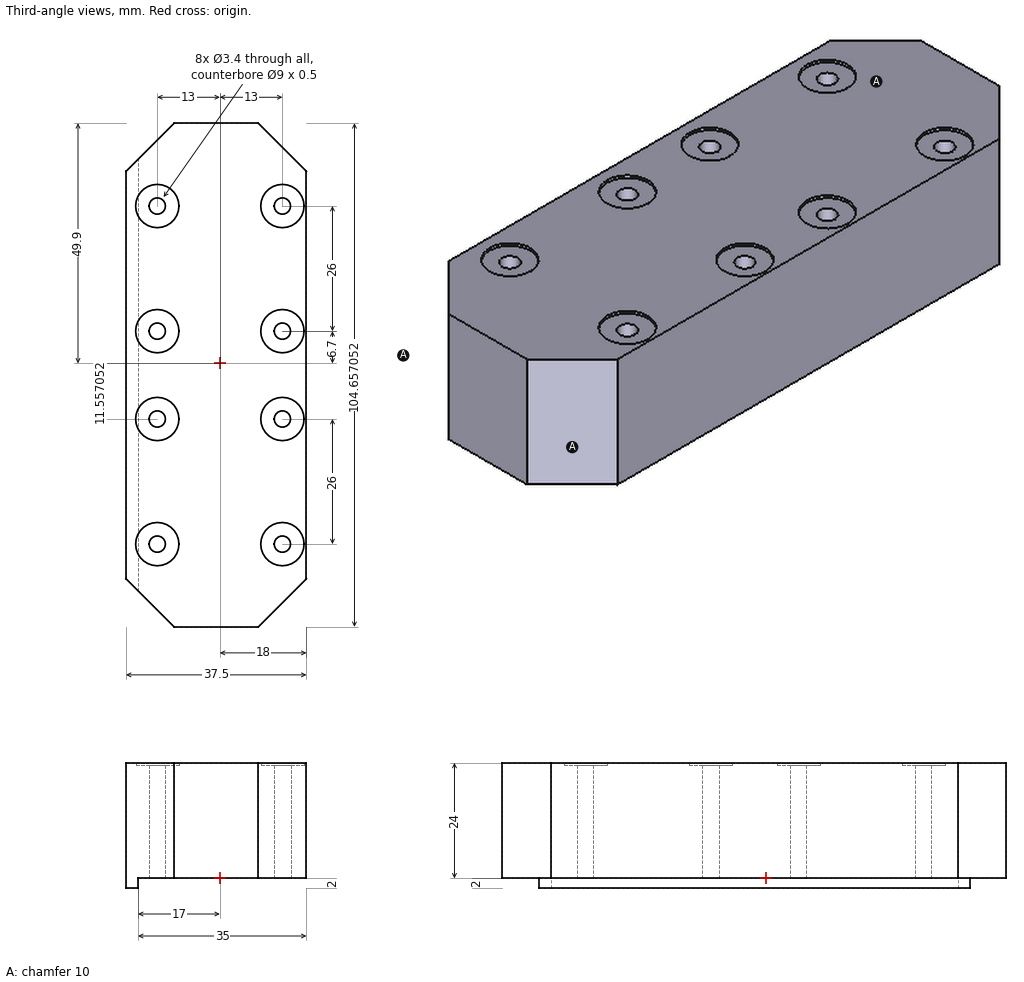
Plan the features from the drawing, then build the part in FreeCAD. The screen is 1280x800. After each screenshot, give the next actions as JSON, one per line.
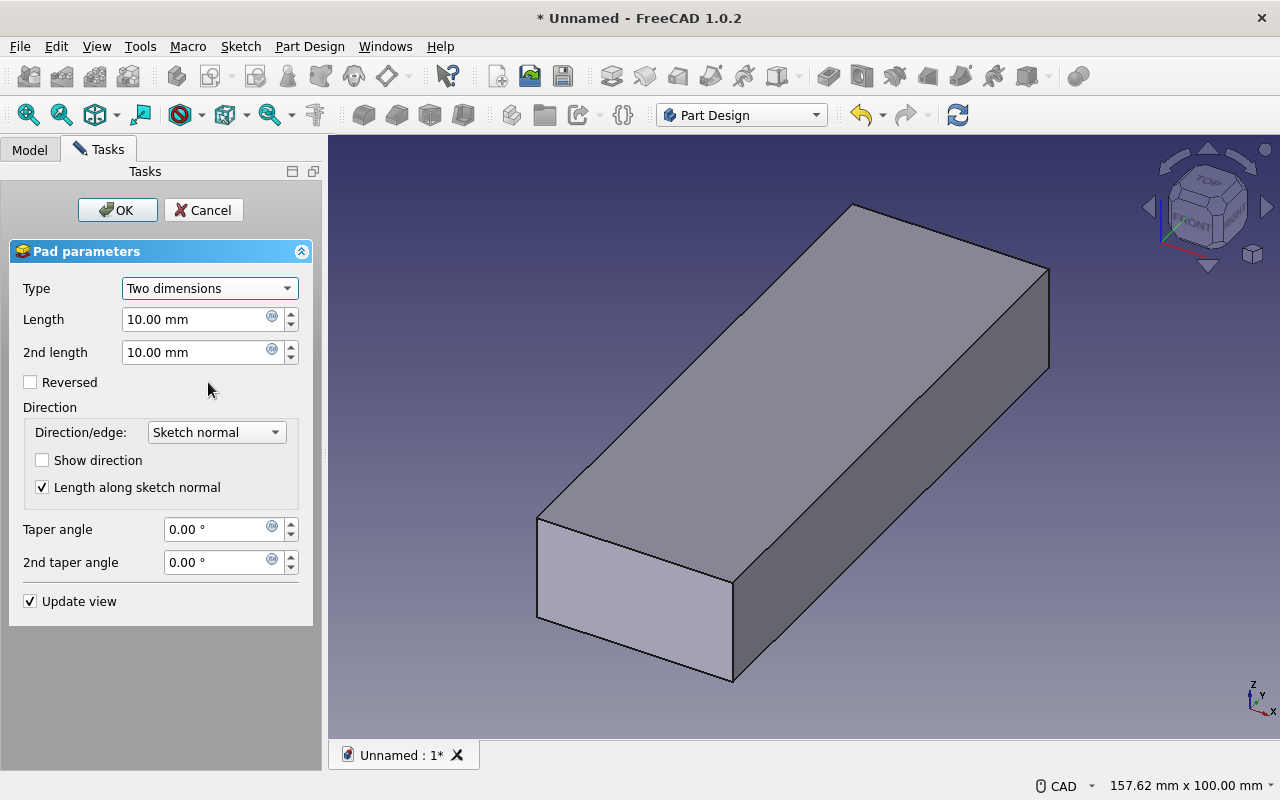
{"action": "triple_click", "coordinate": [204, 320]}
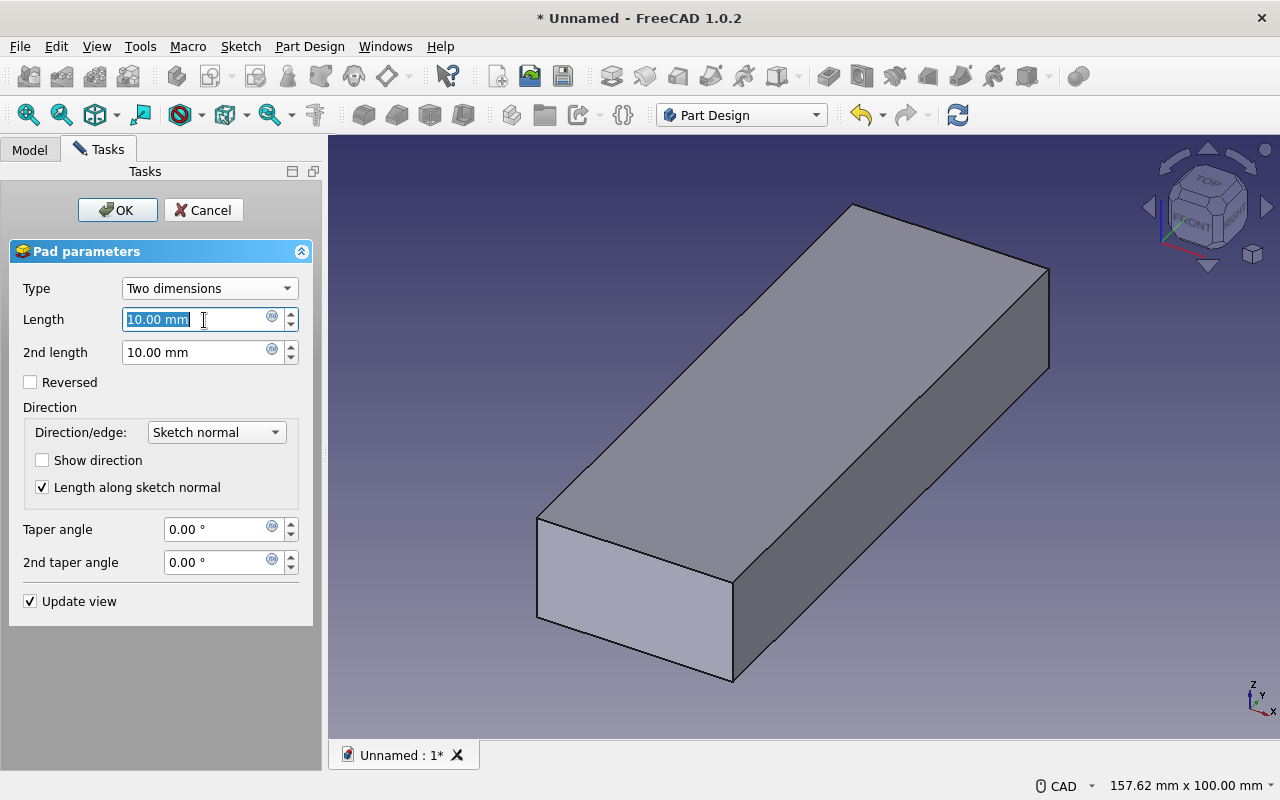
{"action": "type", "text": "24"}
{"action": "key", "text": "Tab"}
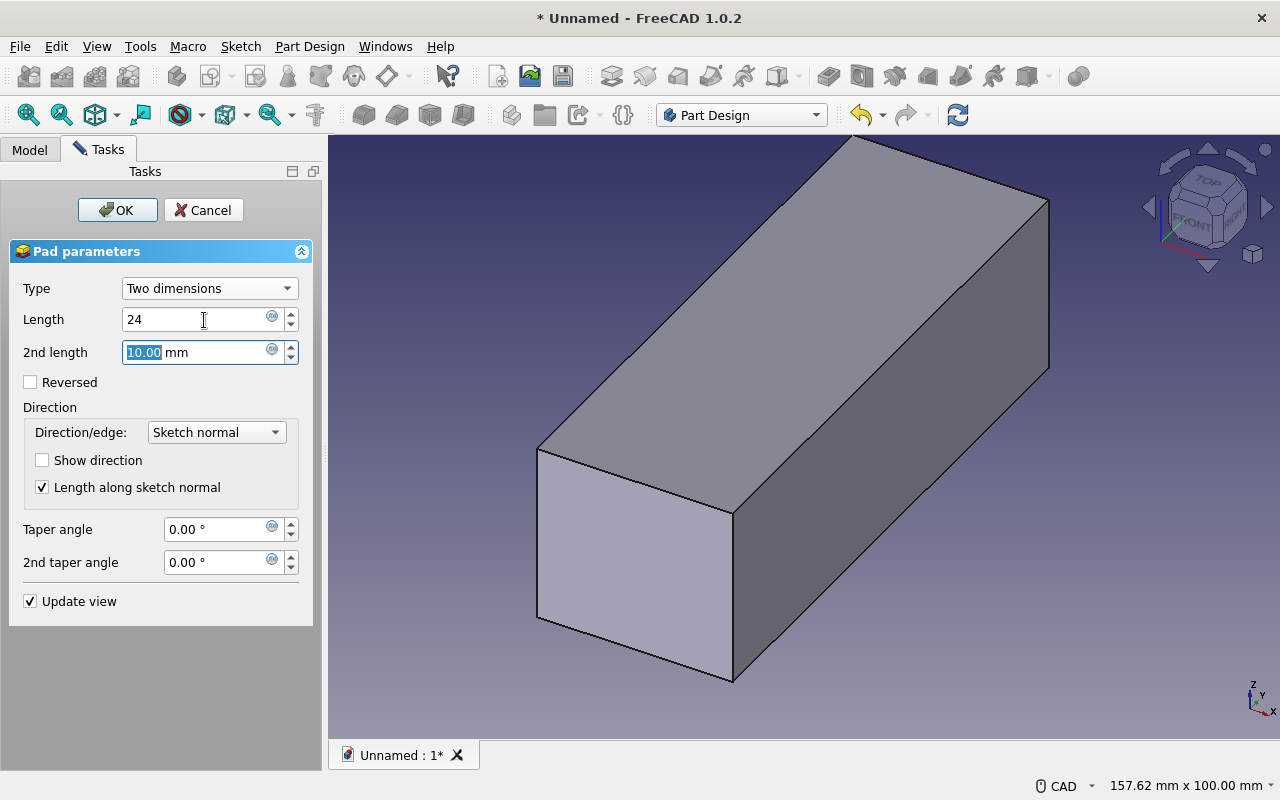
{"action": "type", "text": "2"}
{"action": "key", "text": "Tab"}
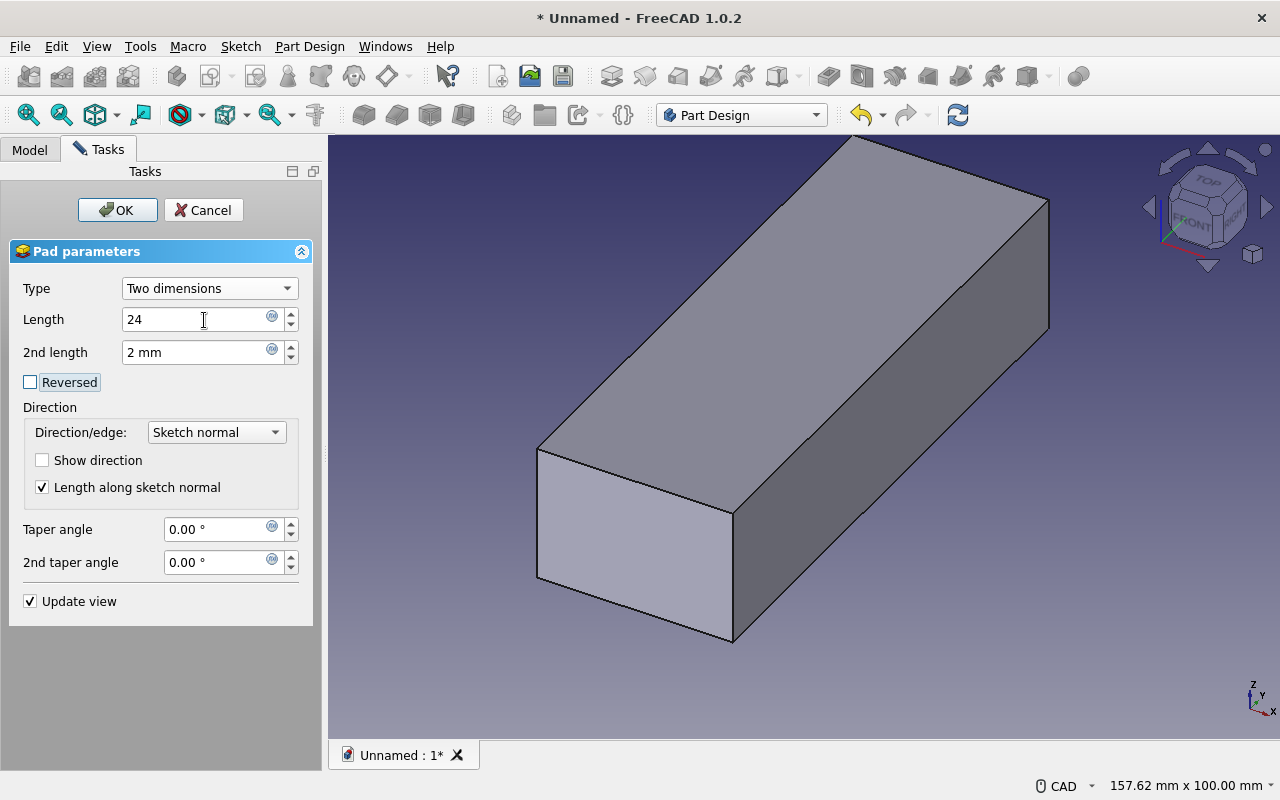
{"action": "left_click", "coordinate": [118, 210]}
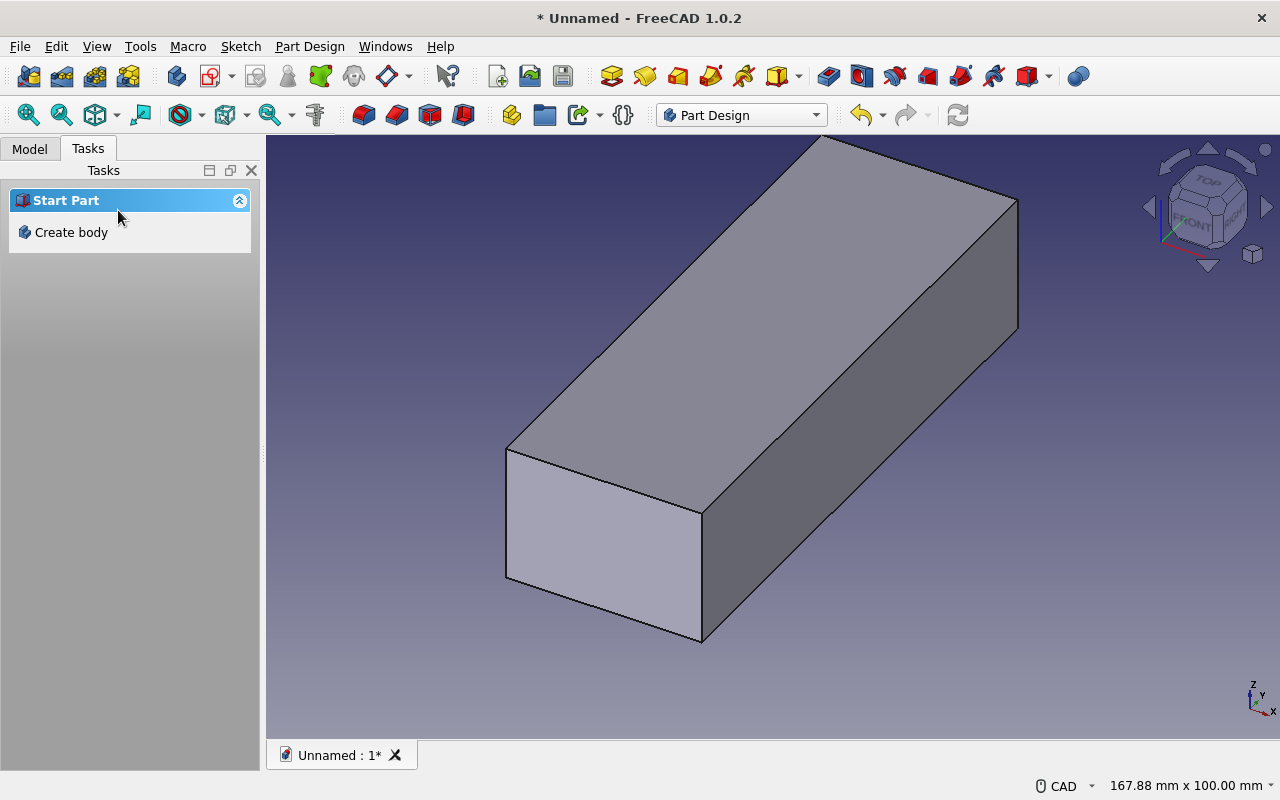
{"action": "left_click", "coordinate": [29, 116]}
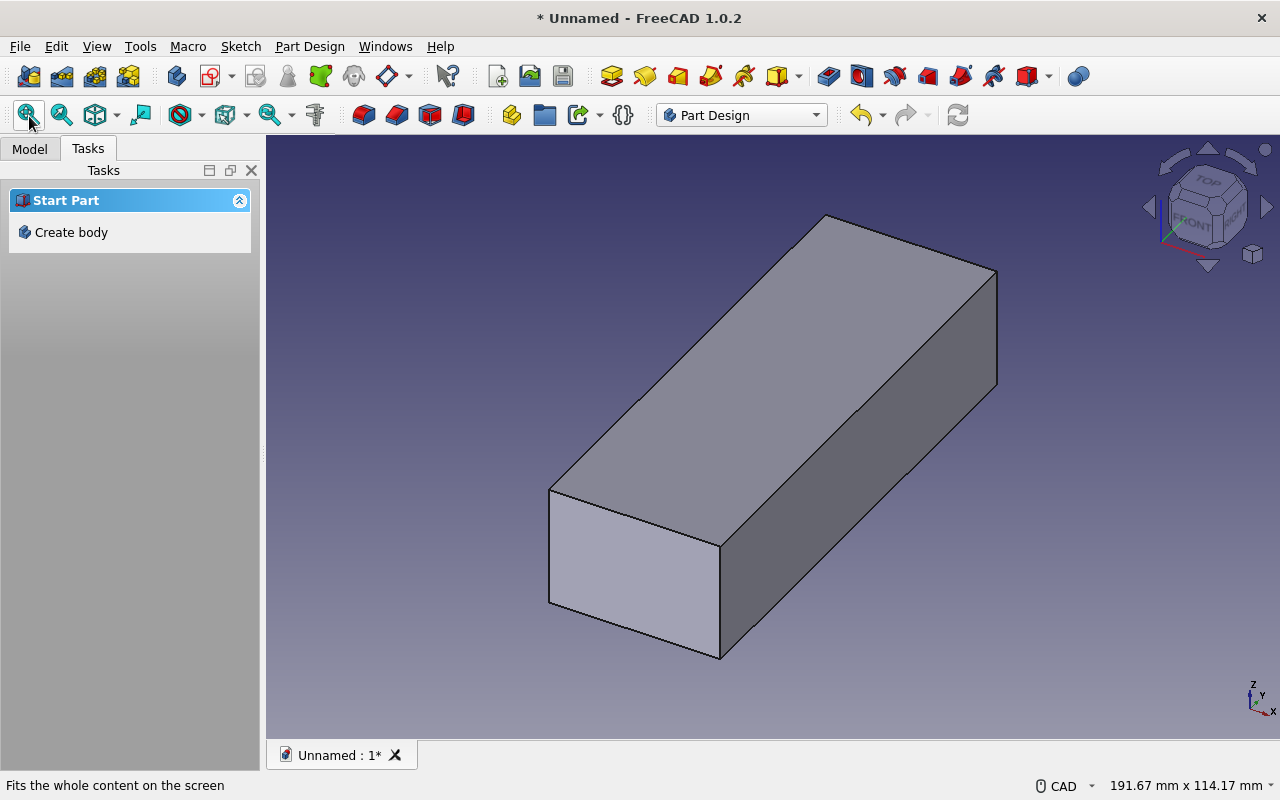
{"action": "left_click", "coordinate": [659, 582]}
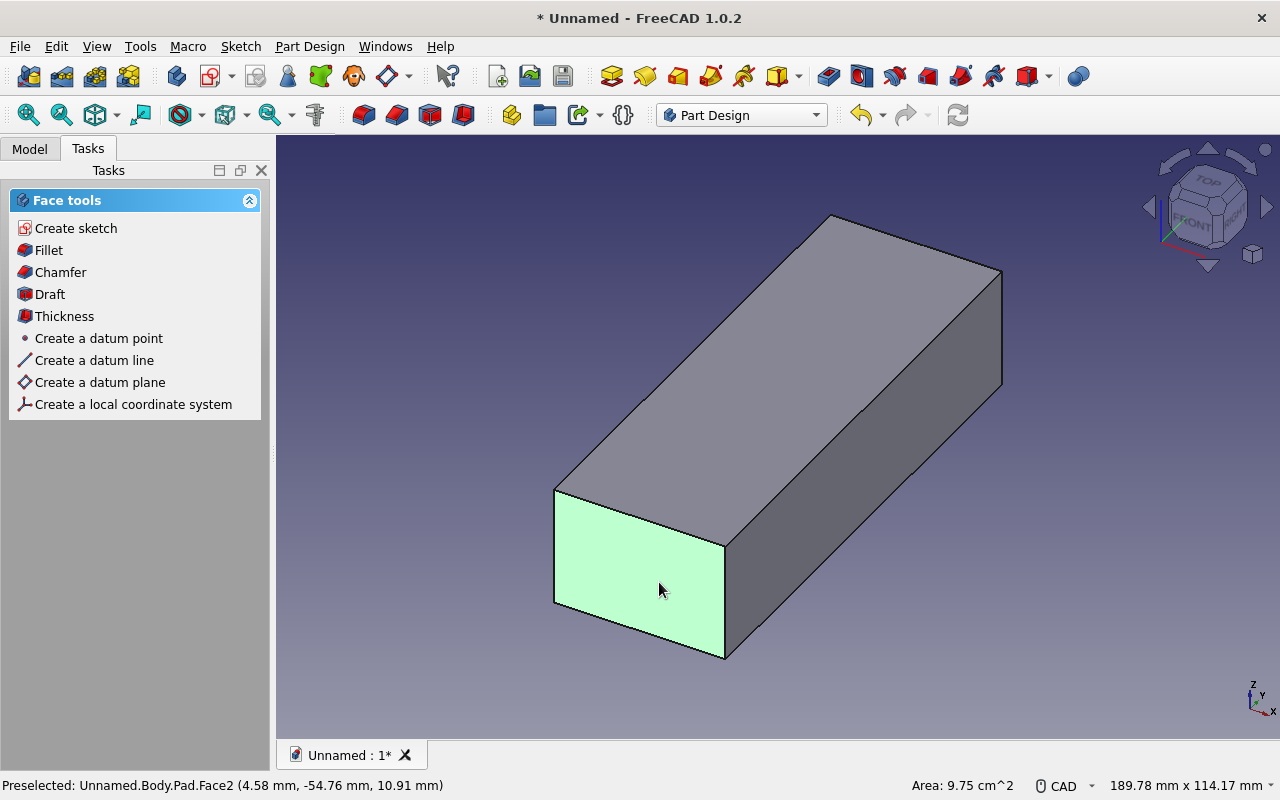
{"action": "left_click", "coordinate": [210, 76]}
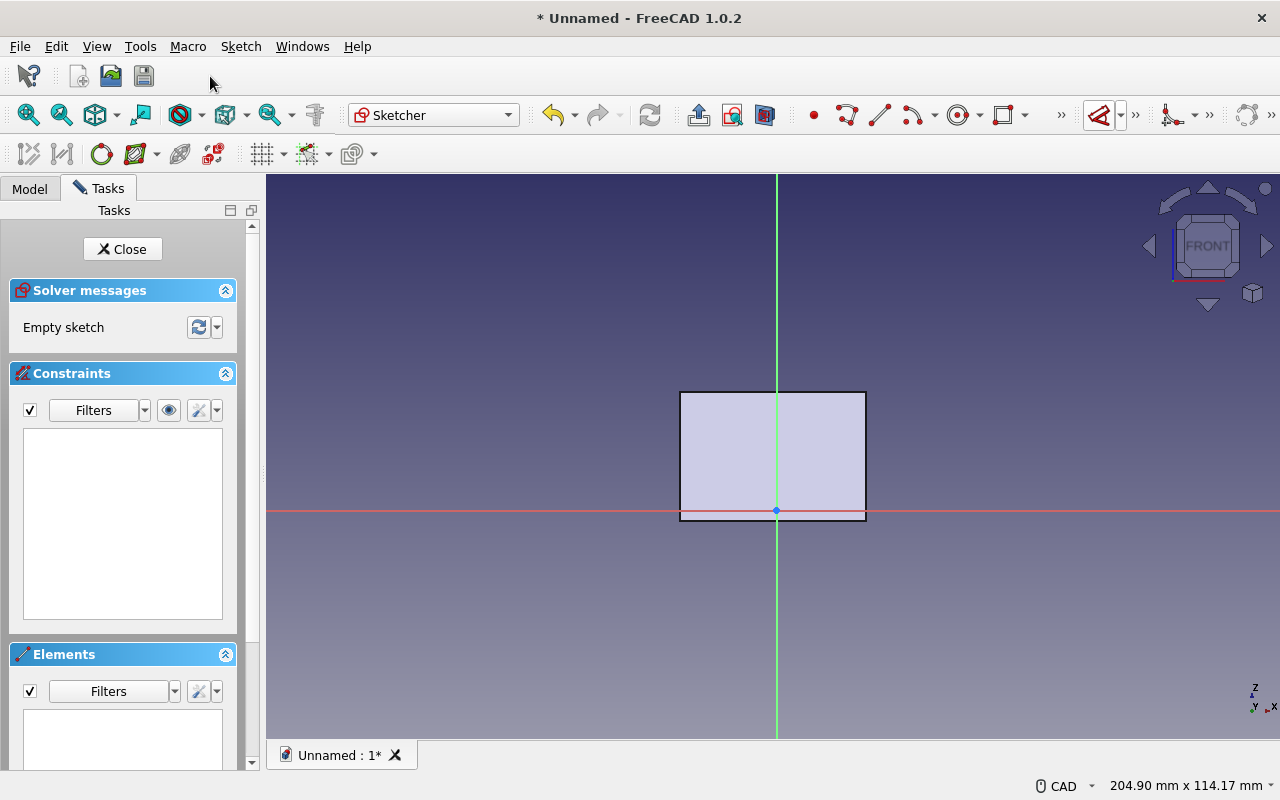
{"action": "scroll", "coordinate": [811, 541], "scroll_direction": "up", "scroll_amount": 6}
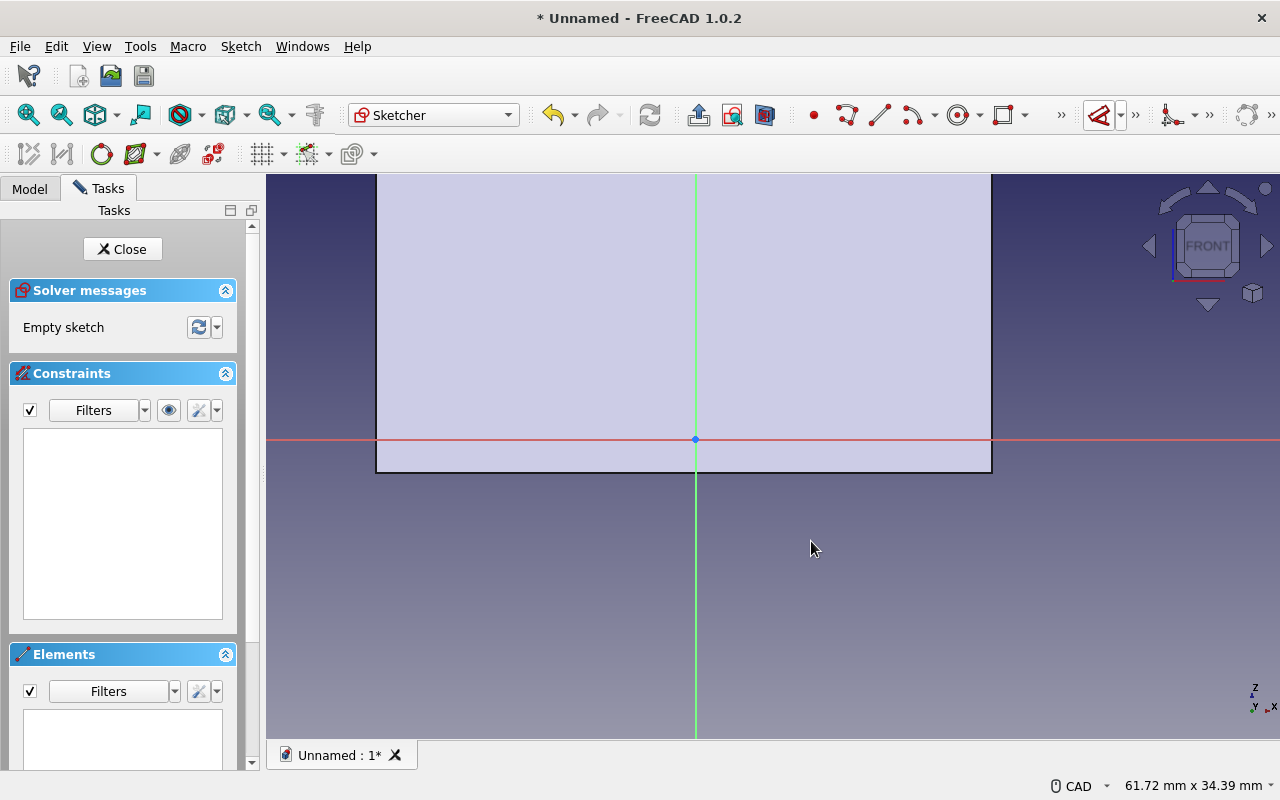
{"action": "left_click", "coordinate": [1002, 116]}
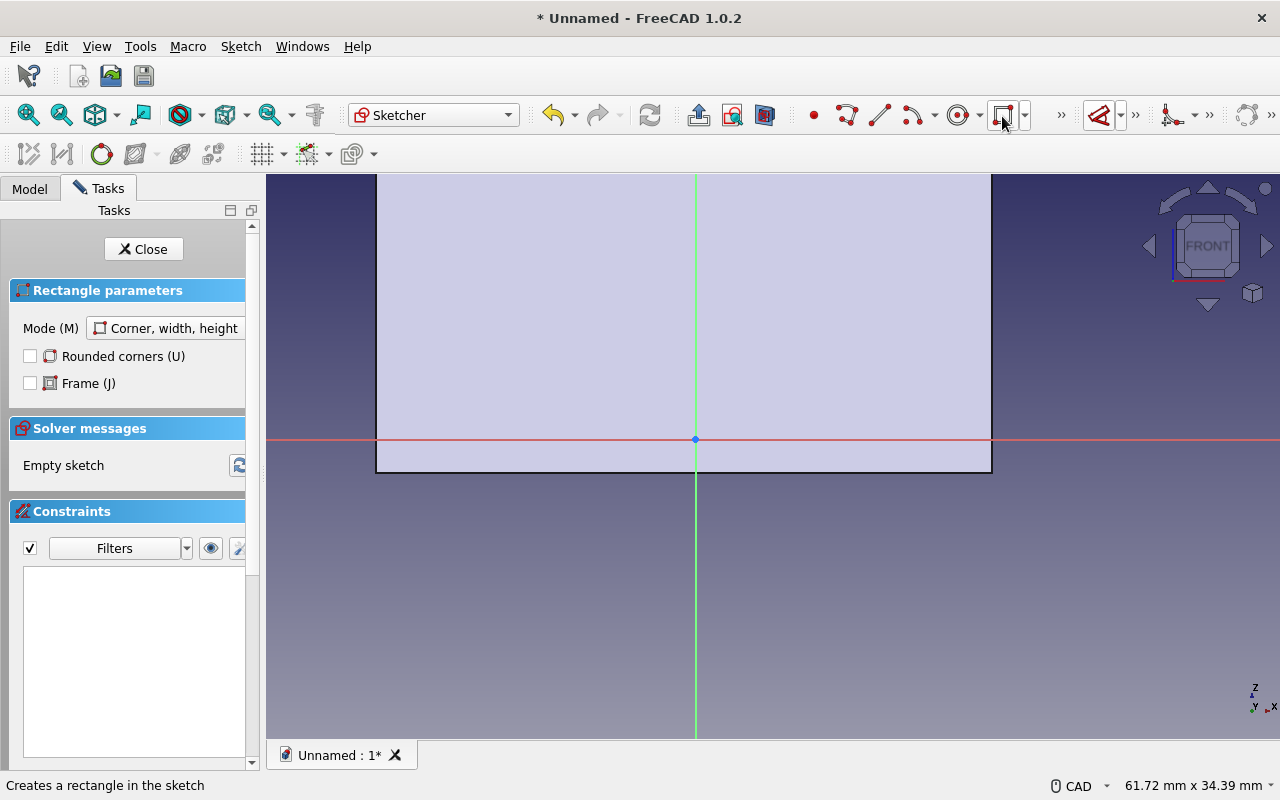
{"action": "left_click", "coordinate": [417, 440]}
{"action": "mouse_move", "coordinate": [992, 473]}